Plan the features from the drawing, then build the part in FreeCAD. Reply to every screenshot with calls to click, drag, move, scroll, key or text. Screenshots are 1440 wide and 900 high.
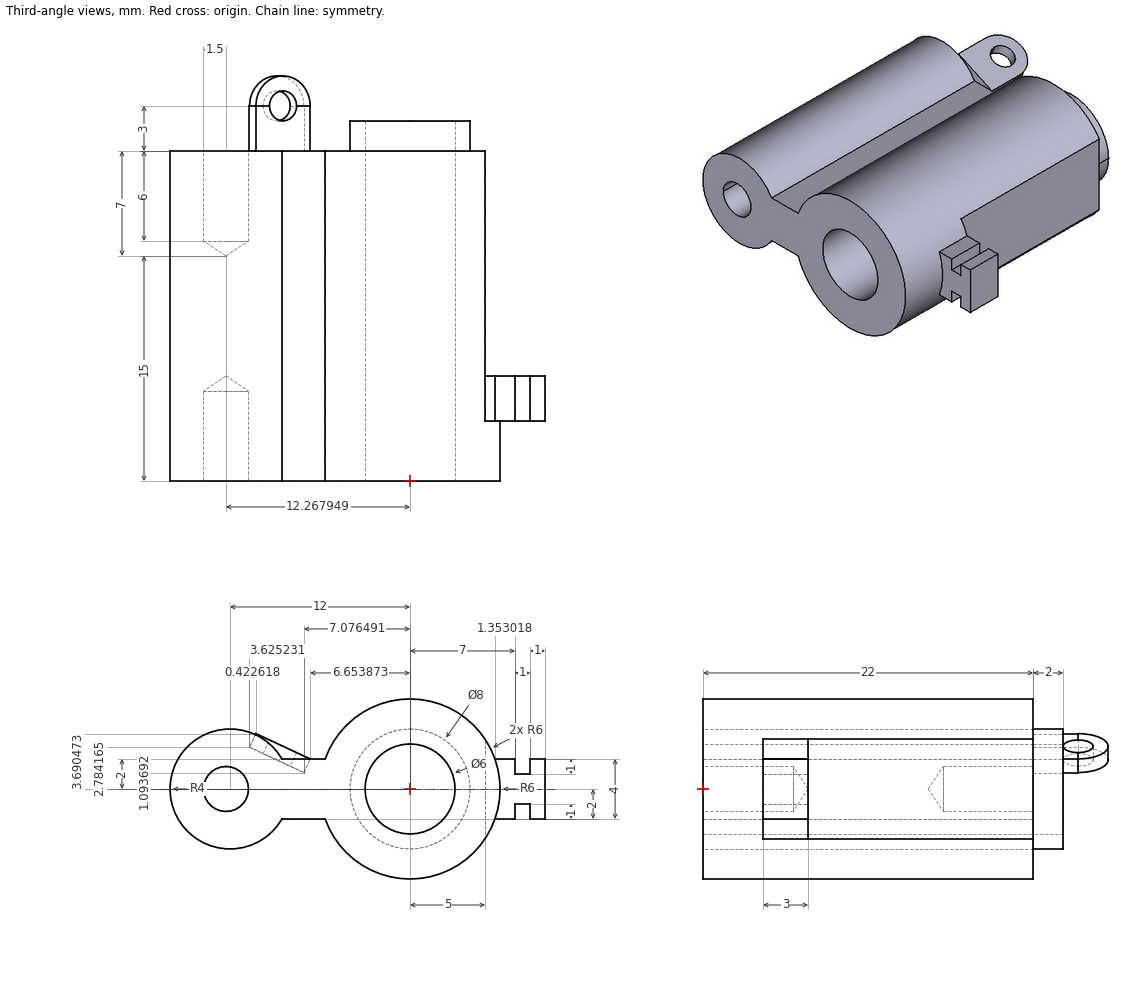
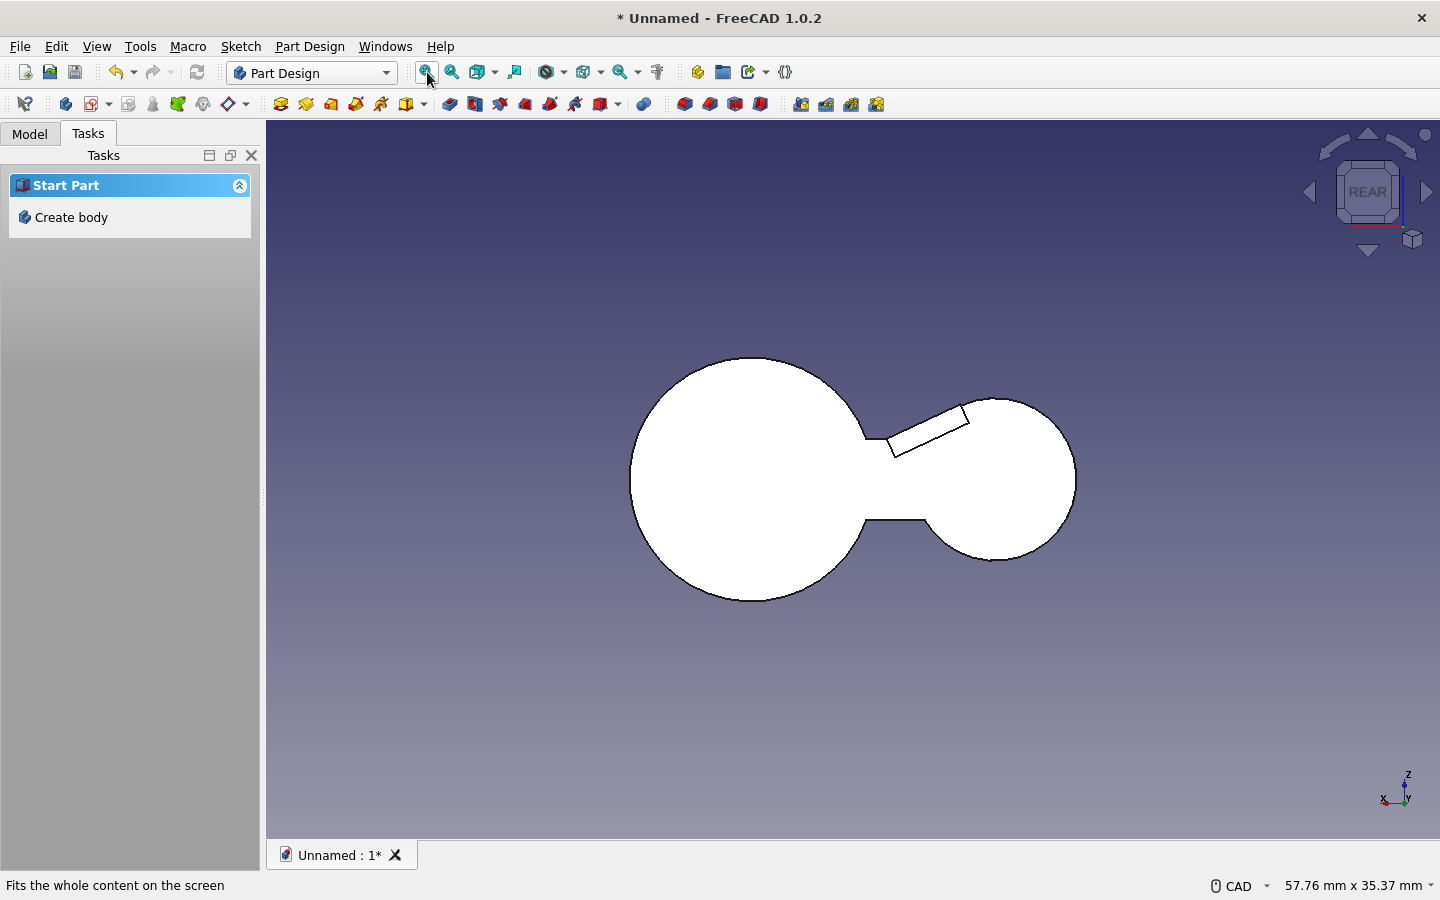
key(0)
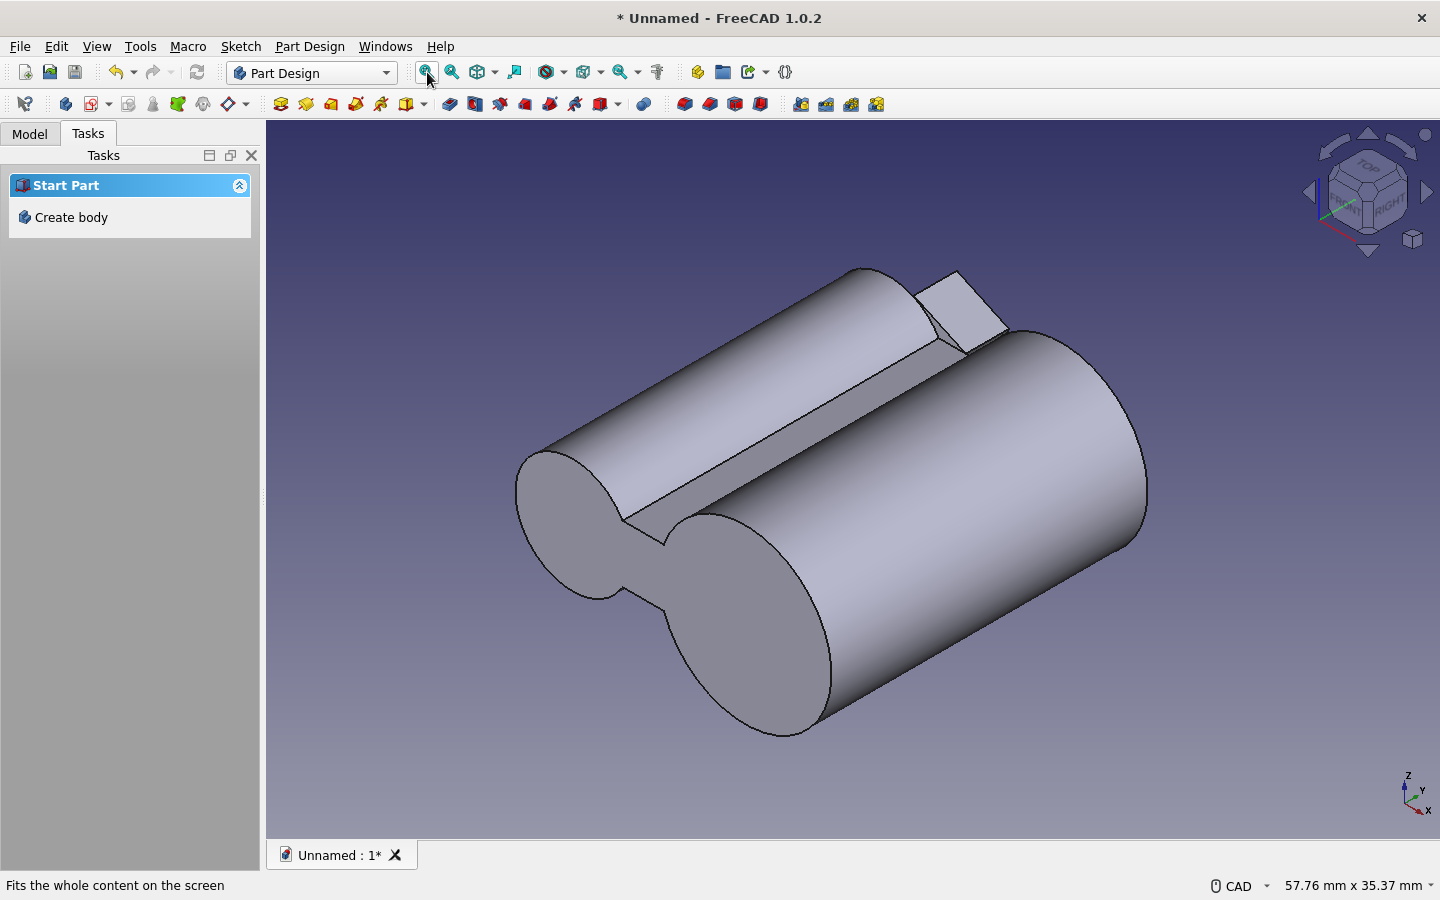
click(961, 311)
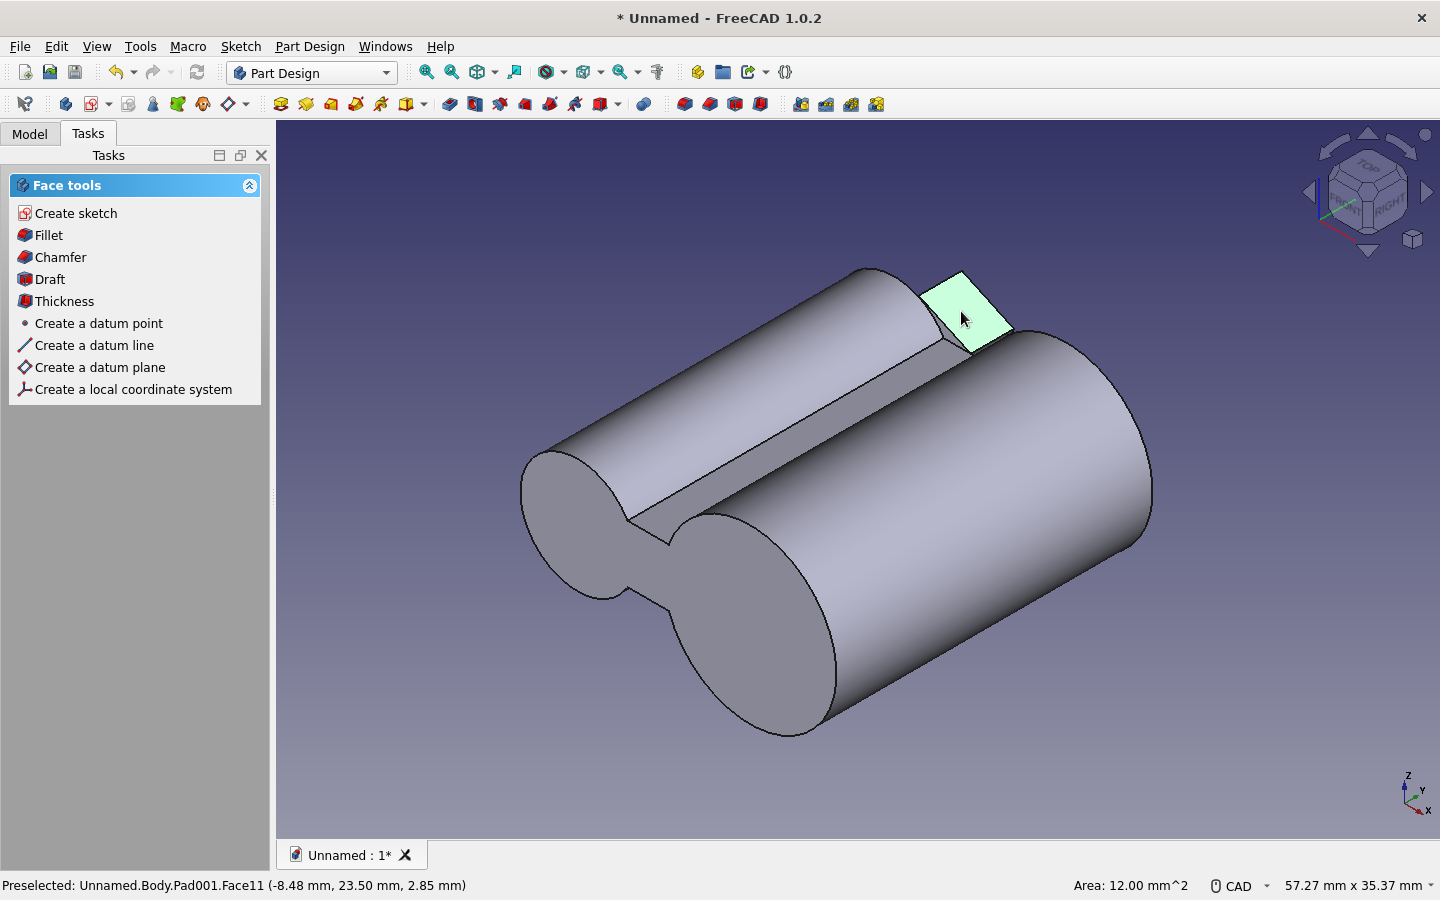
click(90, 104)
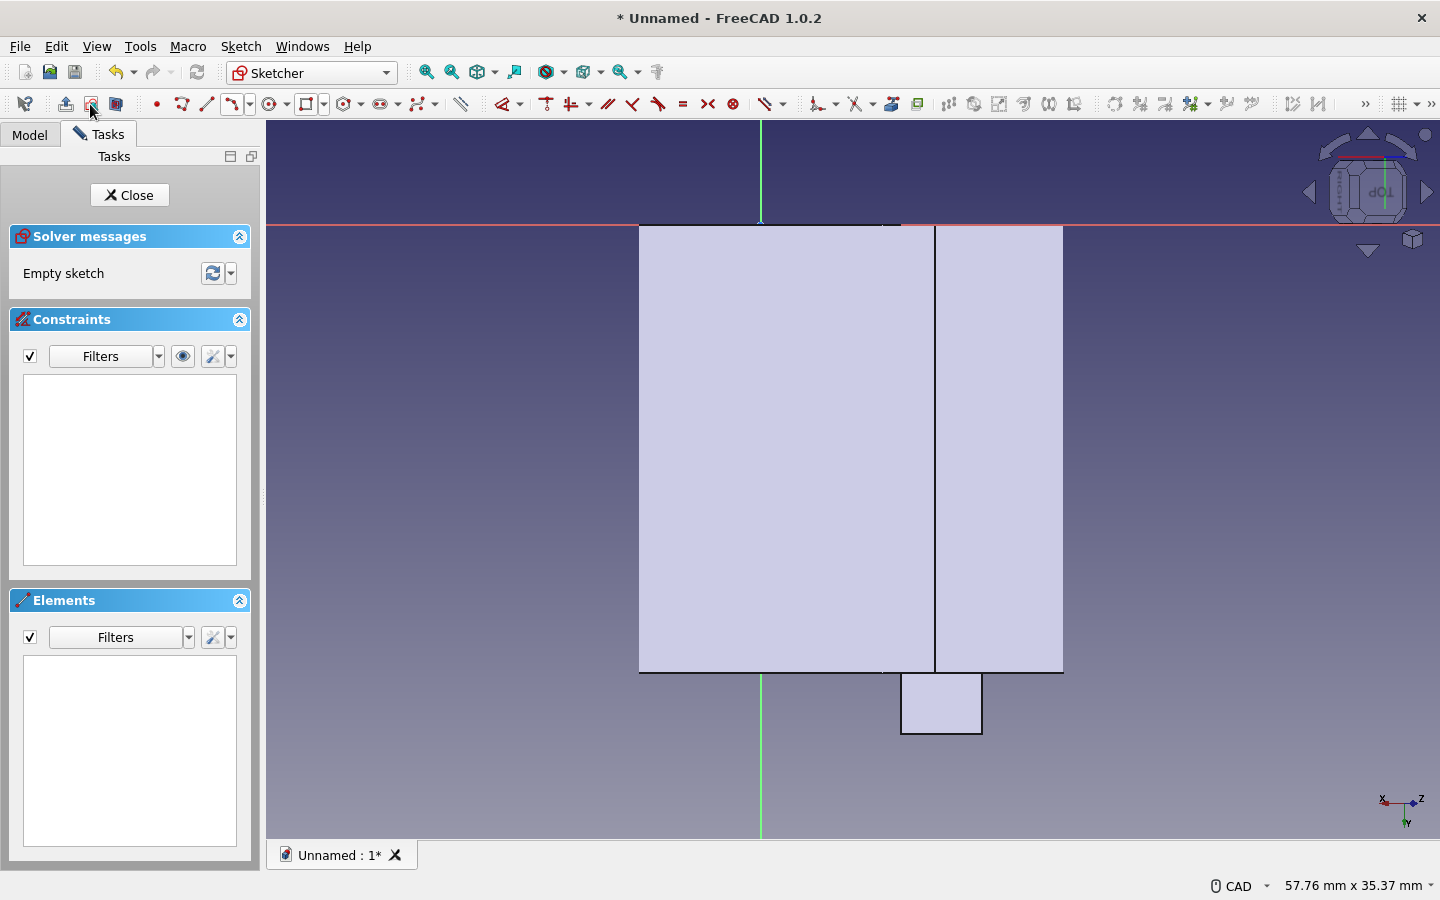
scroll(961, 788, up, 11)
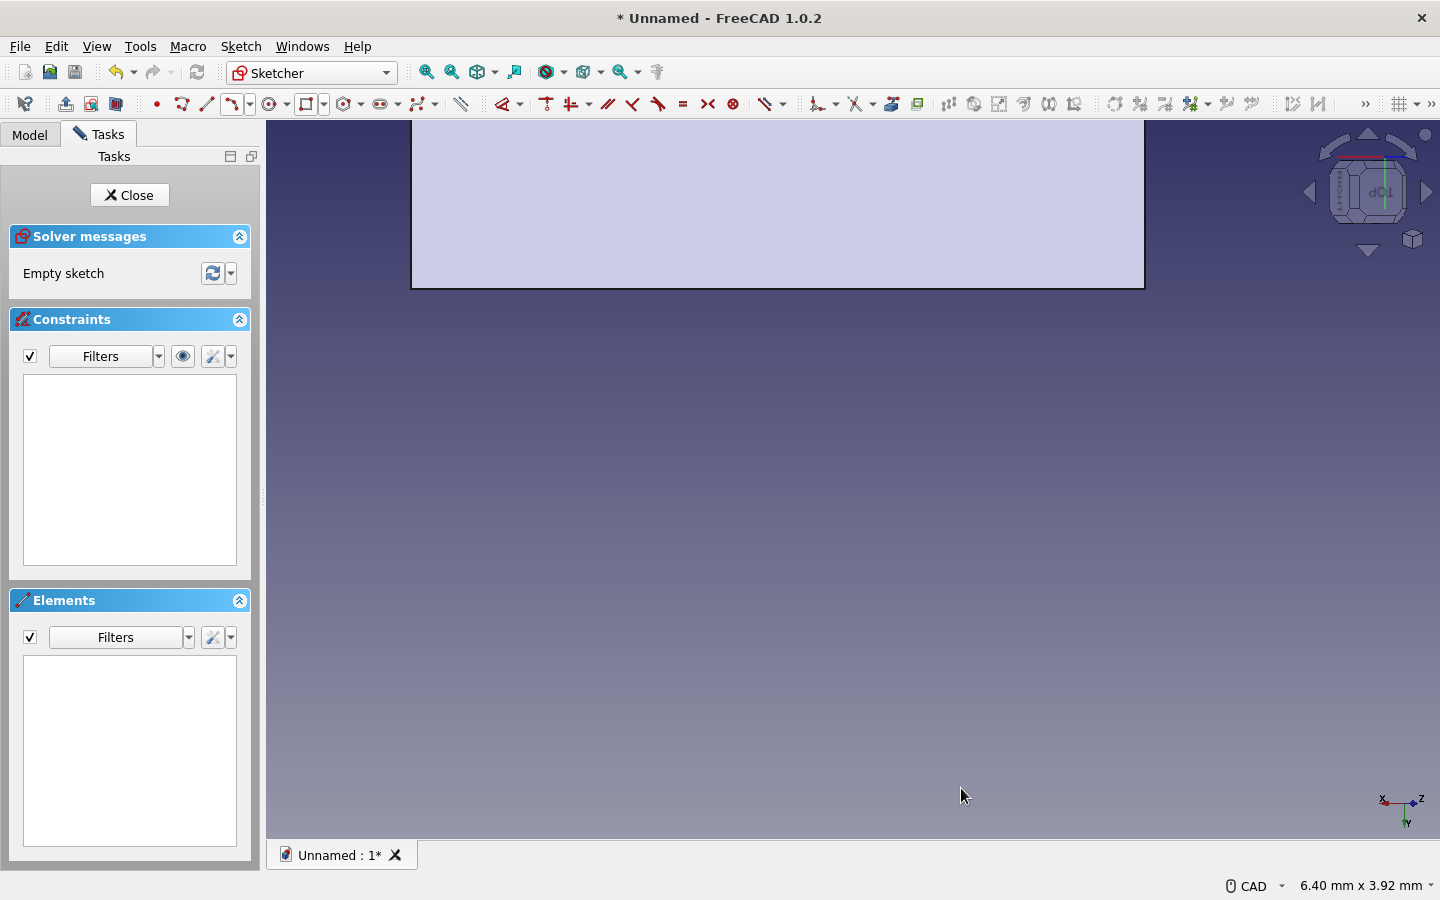
click(207, 104)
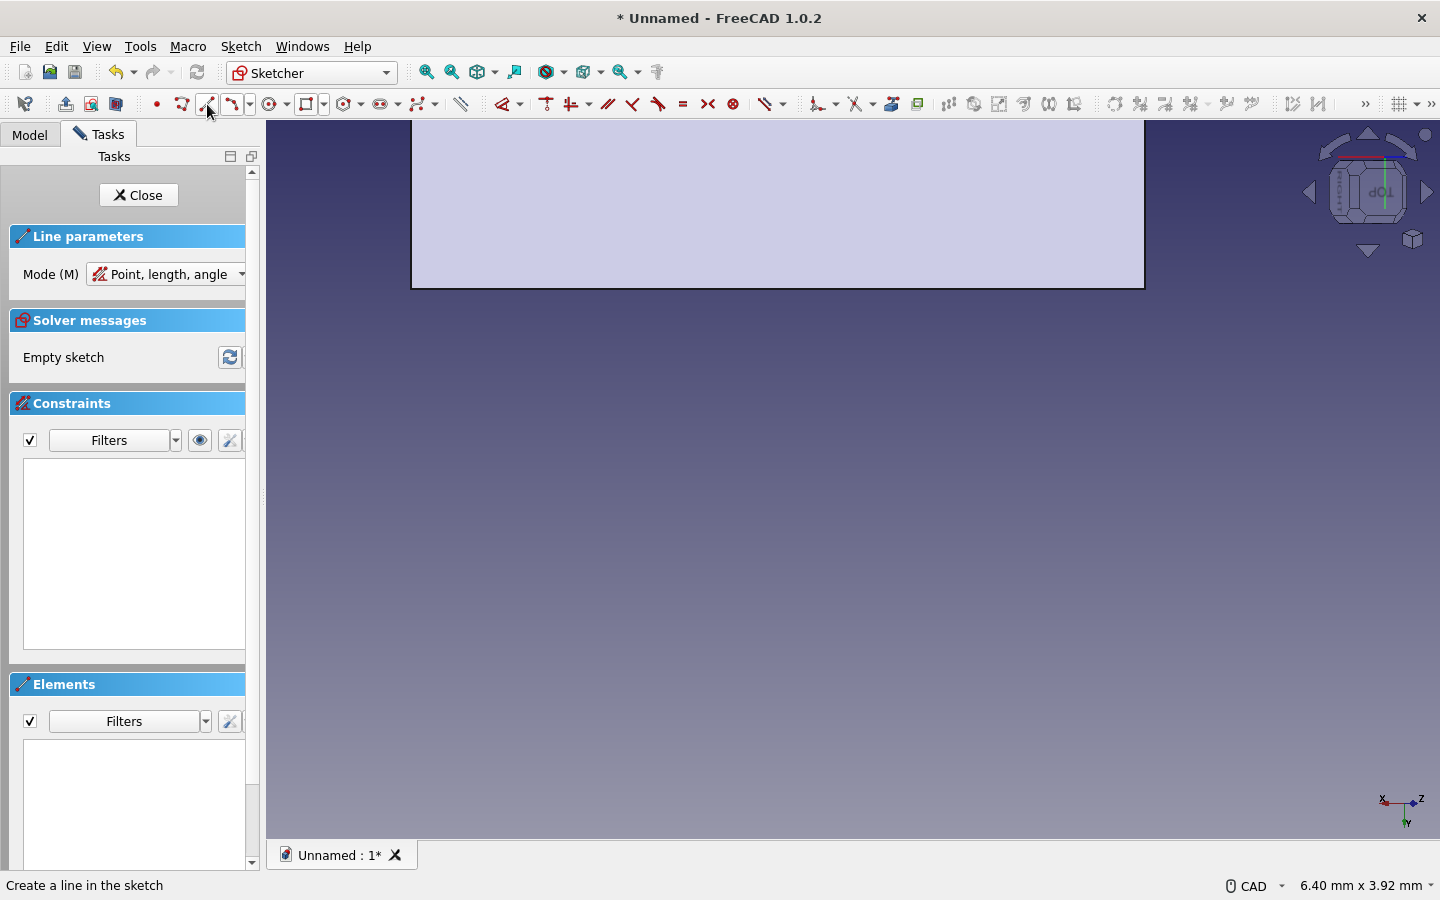
click(1145, 289)
click(411, 289)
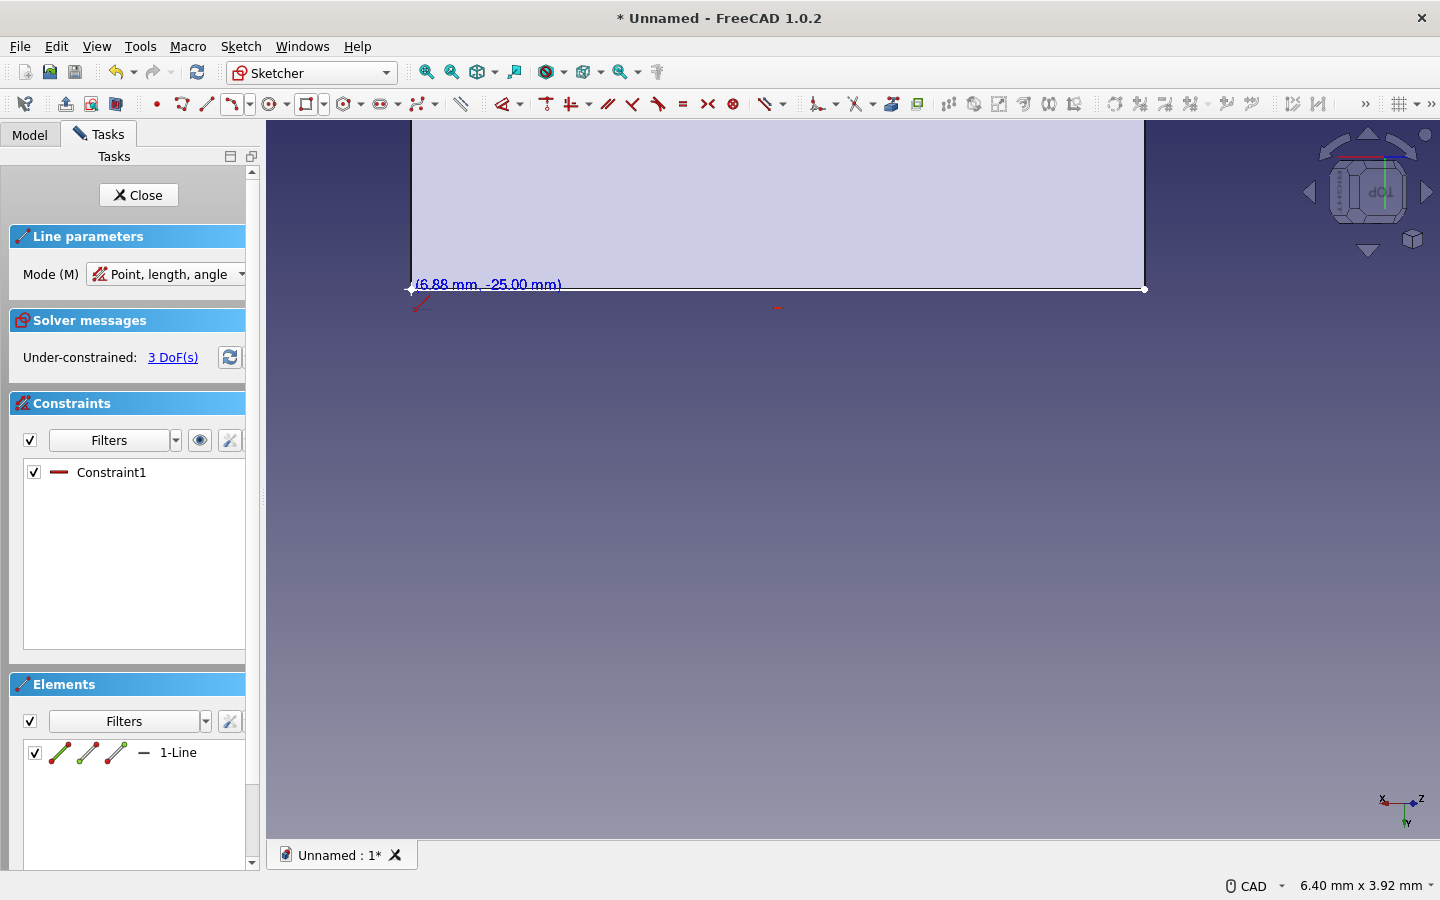
click(232, 104)